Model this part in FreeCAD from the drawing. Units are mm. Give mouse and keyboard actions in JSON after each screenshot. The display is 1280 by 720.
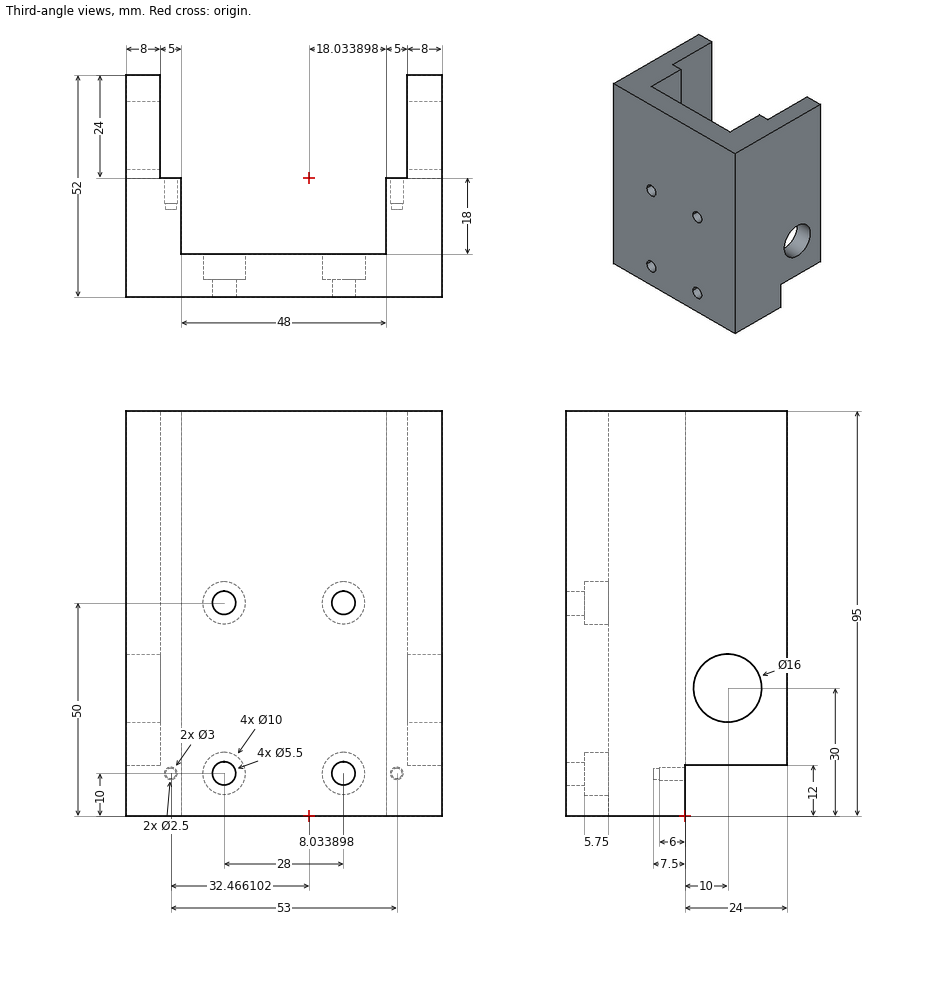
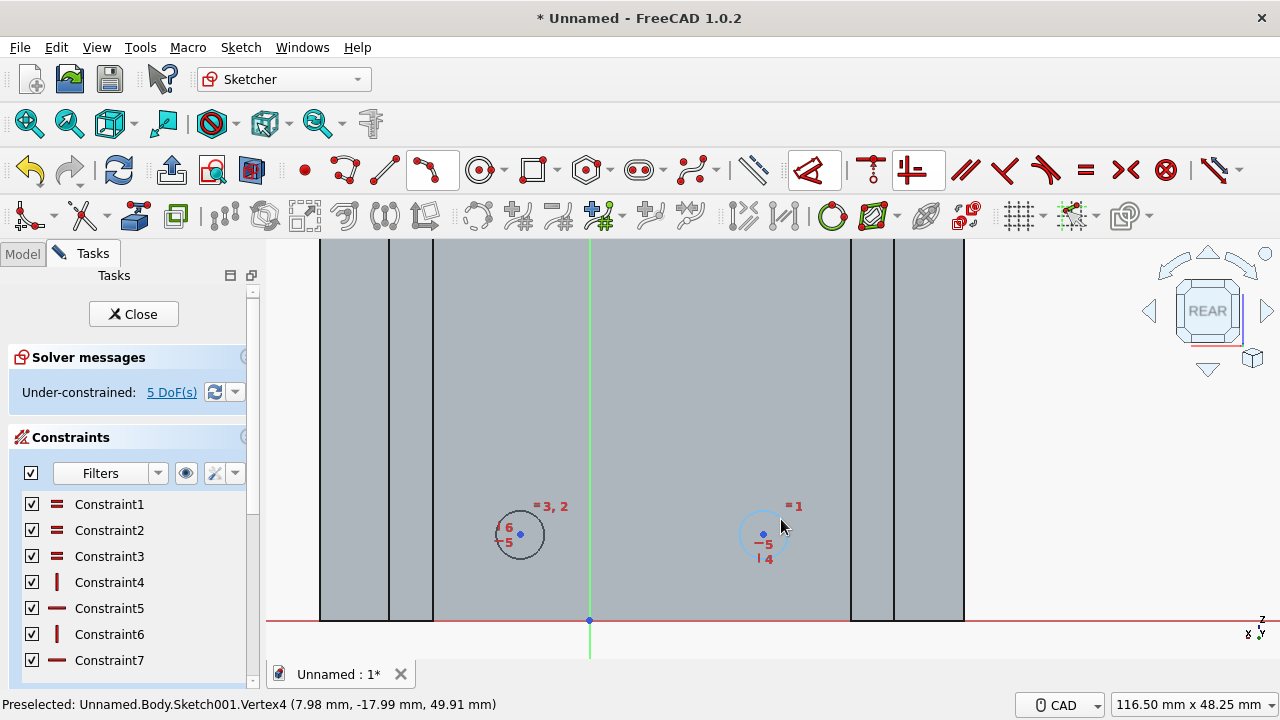
{"action": "left_click", "coordinate": [781, 518]}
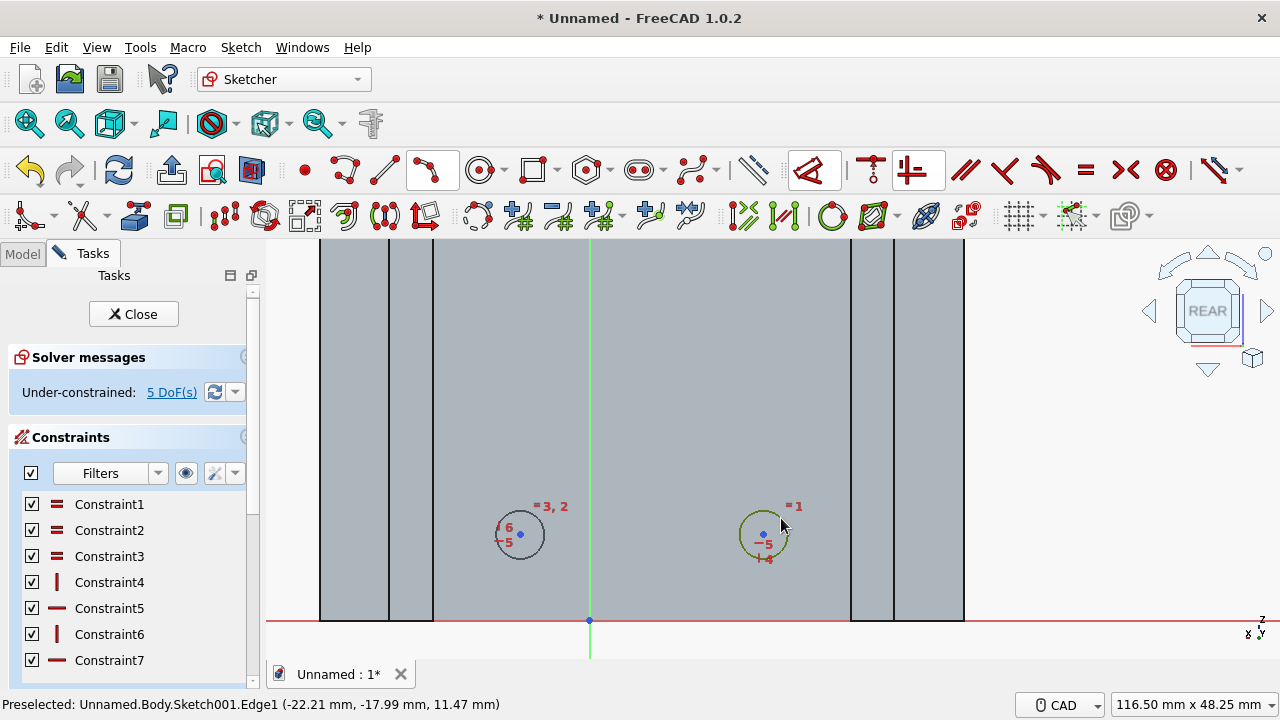
{"action": "key", "text": "k o"}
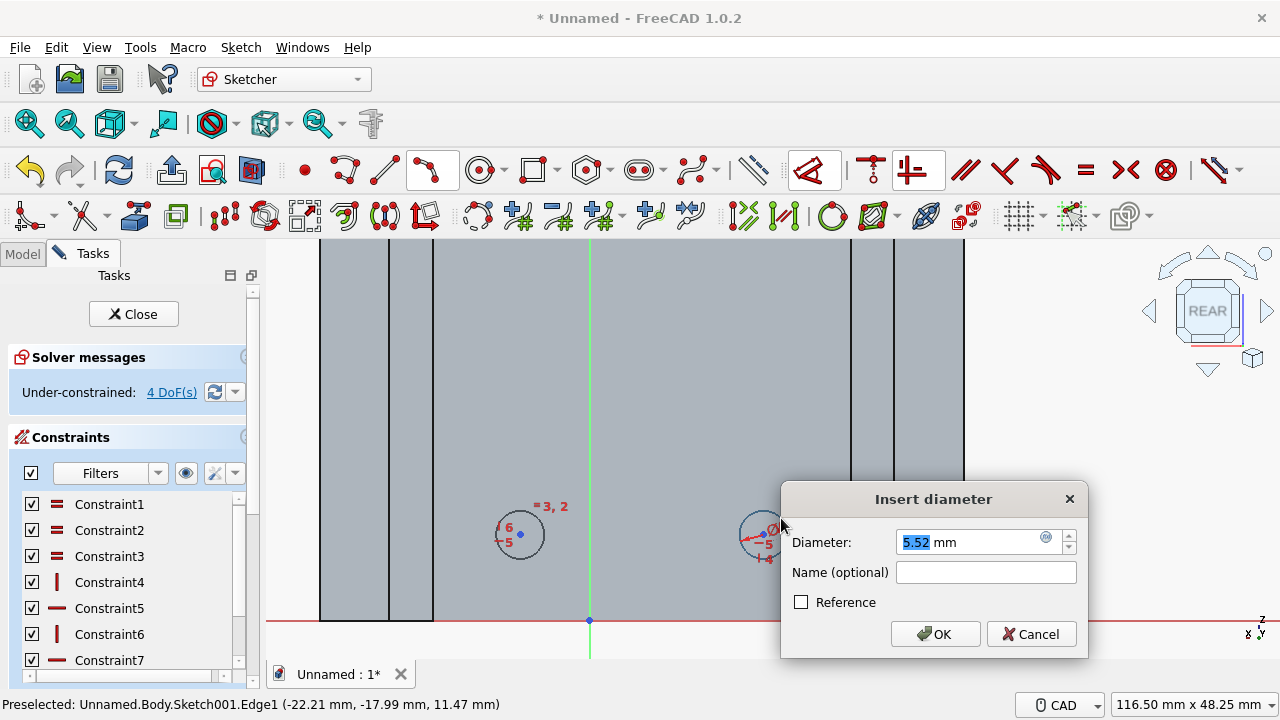
{"action": "type", "text": "5.5"}
{"action": "key", "text": "Return"}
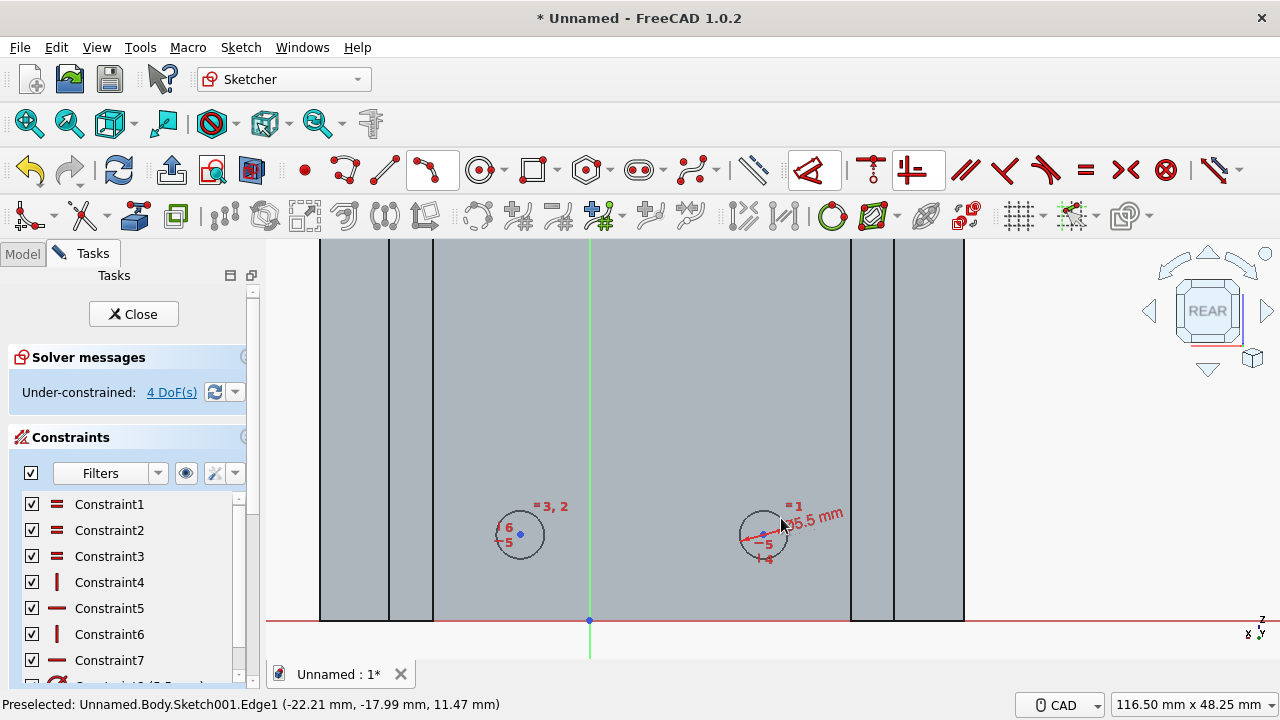
{"action": "left_click", "coordinate": [764, 535]}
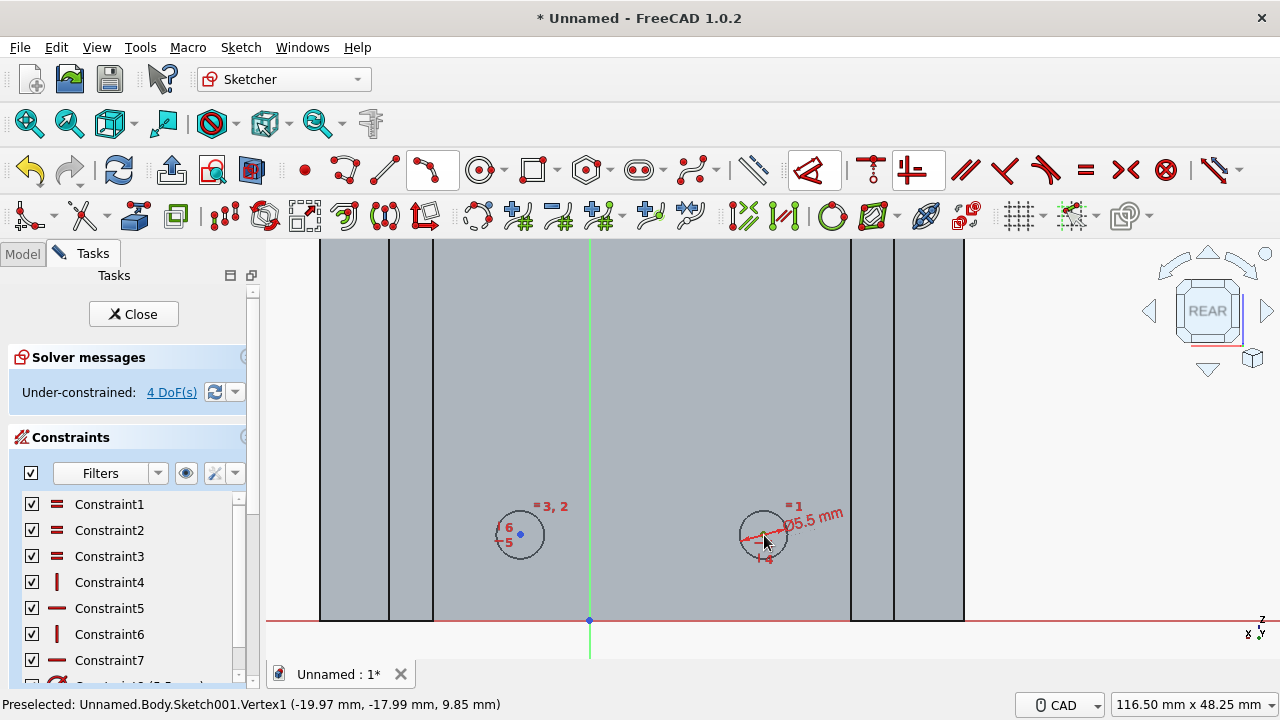
{"action": "key", "text": "i"}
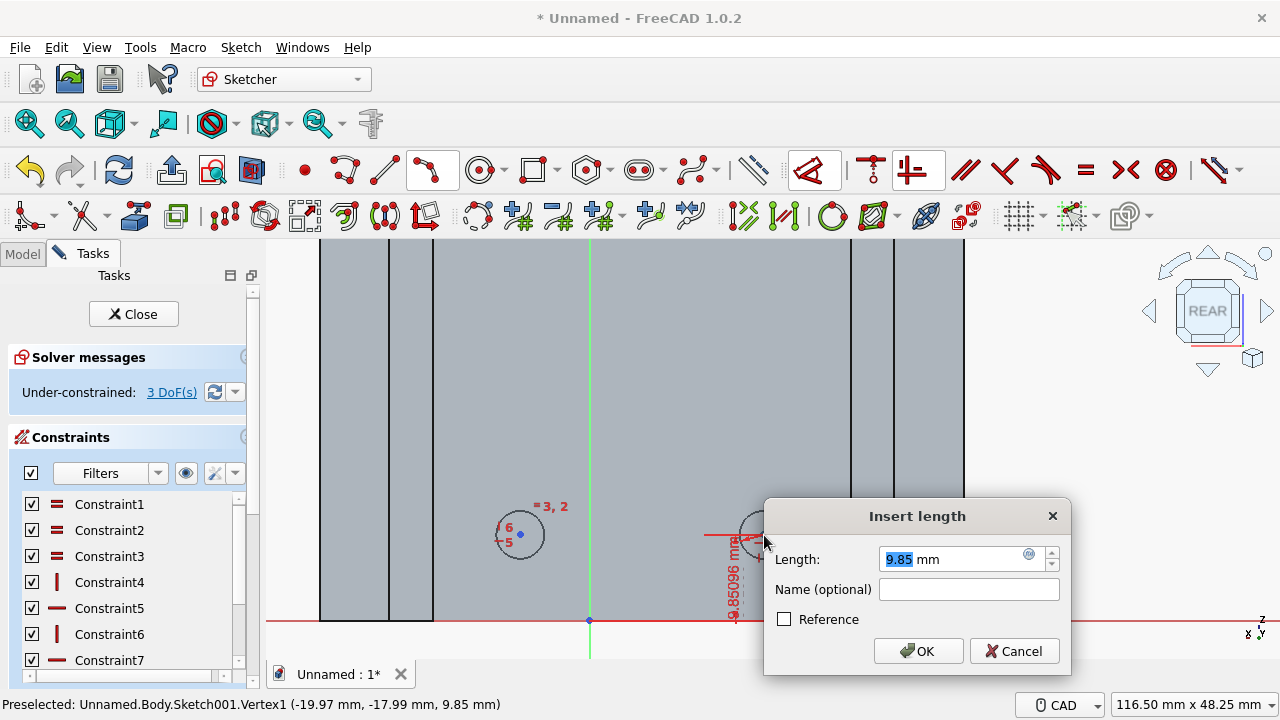
{"action": "type", "text": "10"}
{"action": "key", "text": "Return"}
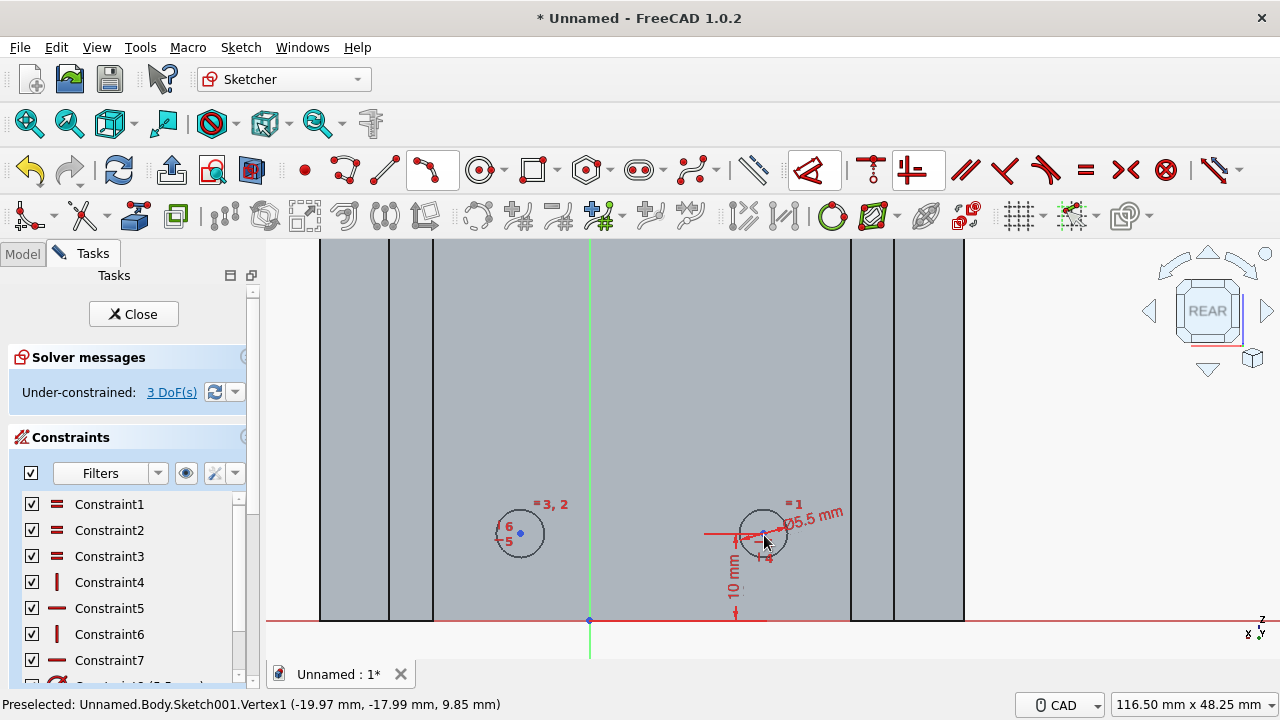
{"action": "scroll", "coordinate": [781, 519], "scroll_direction": "down", "scroll_amount": 3}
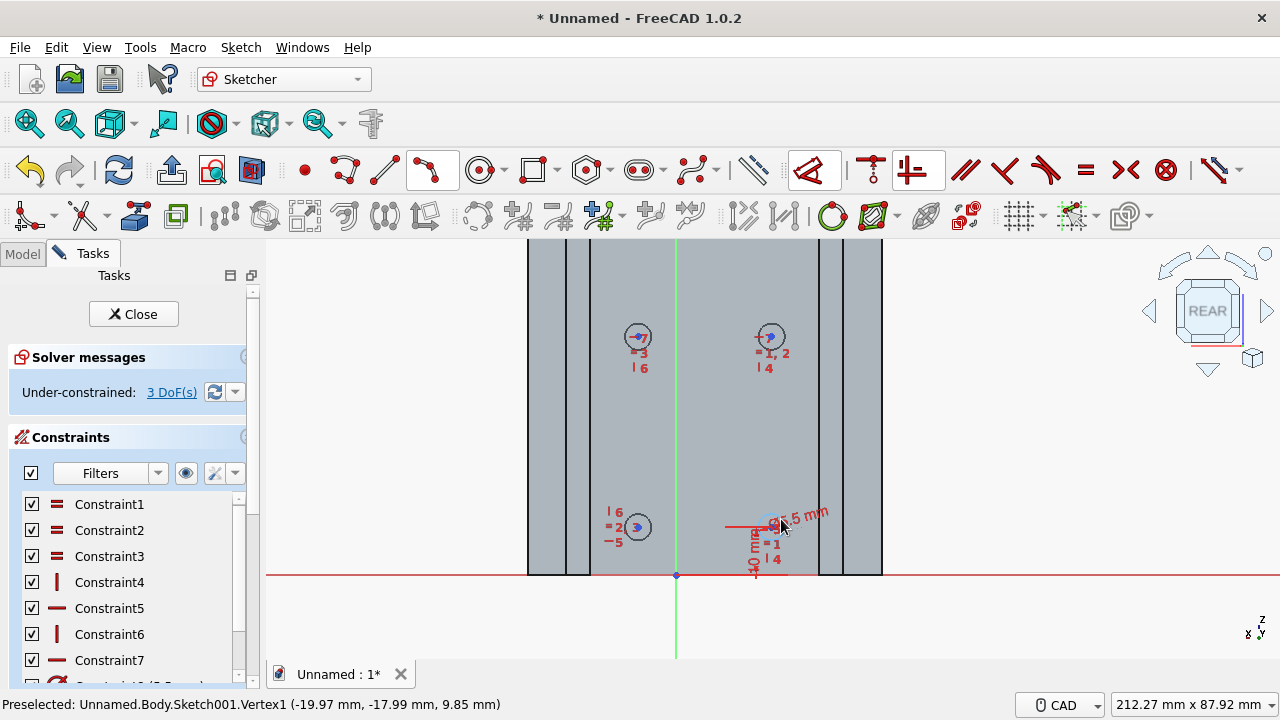
{"action": "left_click", "coordinate": [772, 337]}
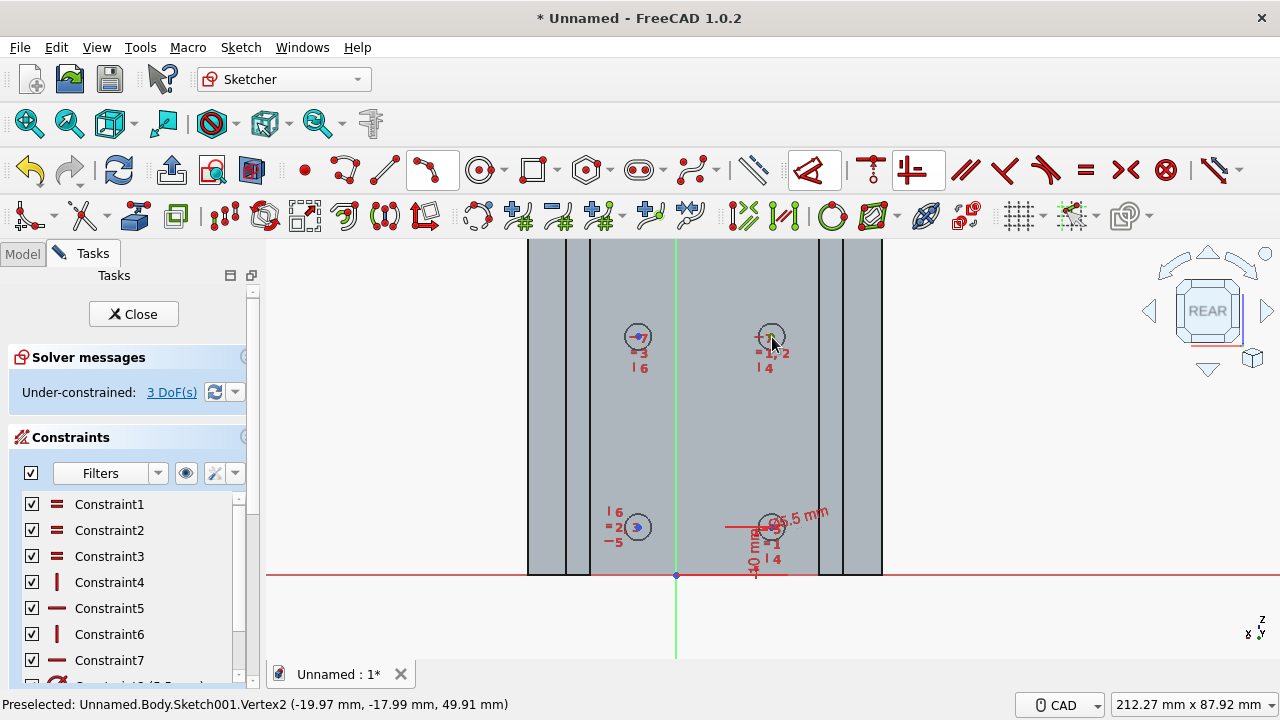
{"action": "key", "text": "i"}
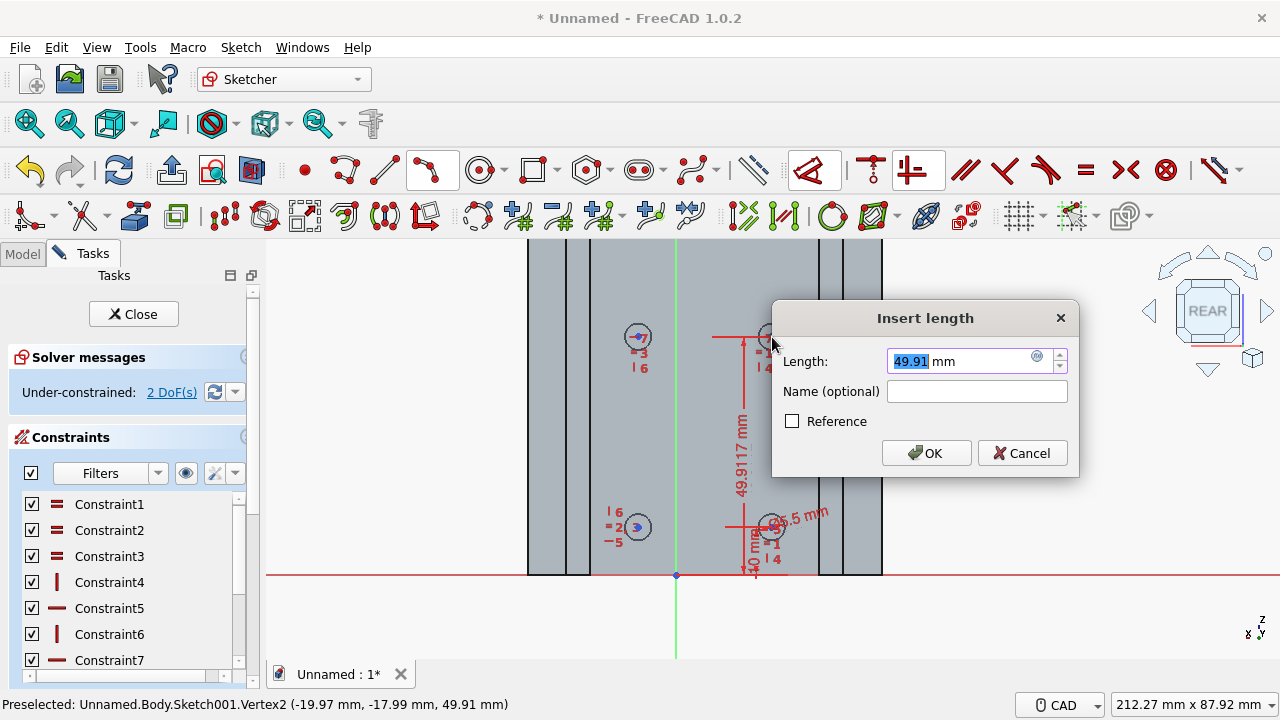
{"action": "type", "text": "50"}
{"action": "key", "text": "Return"}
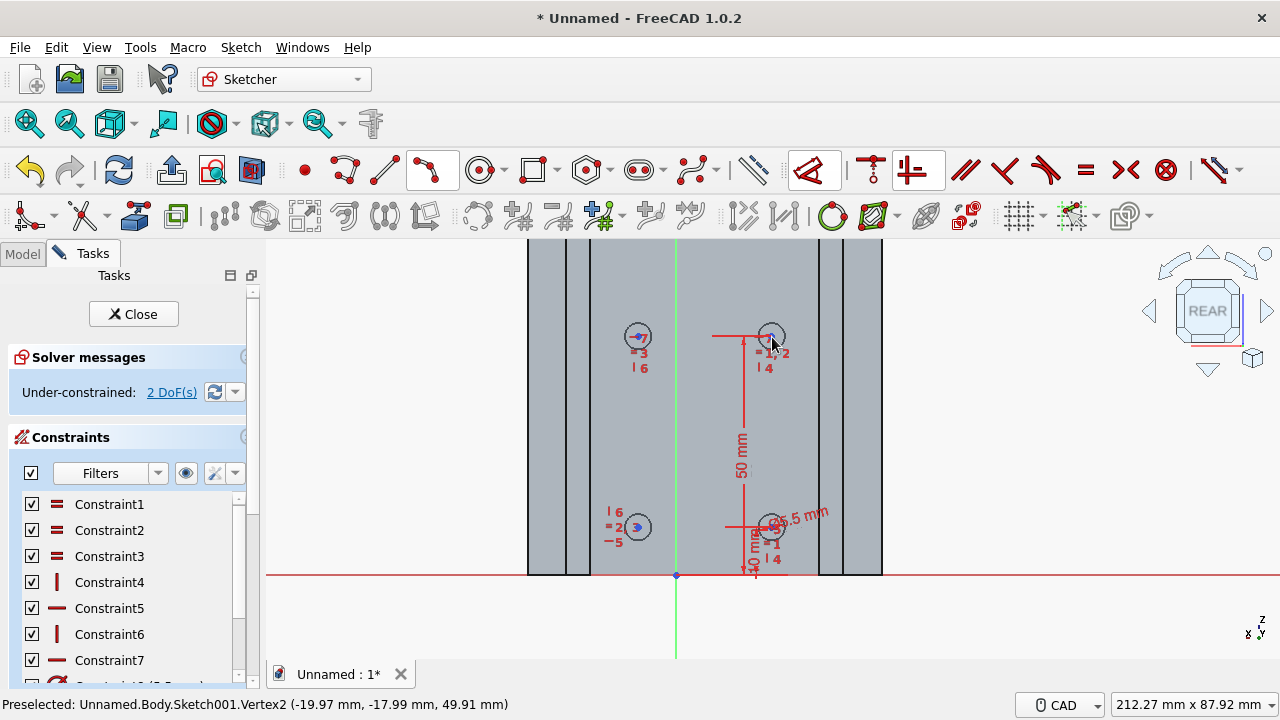
{"action": "left_click", "coordinate": [772, 527]}